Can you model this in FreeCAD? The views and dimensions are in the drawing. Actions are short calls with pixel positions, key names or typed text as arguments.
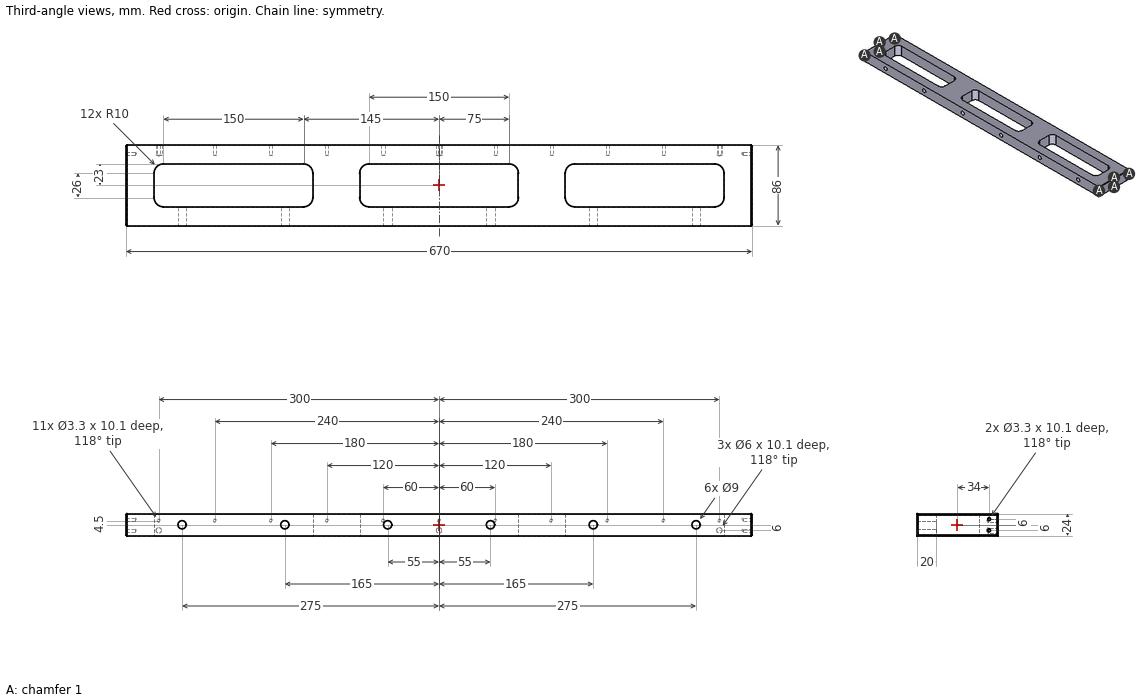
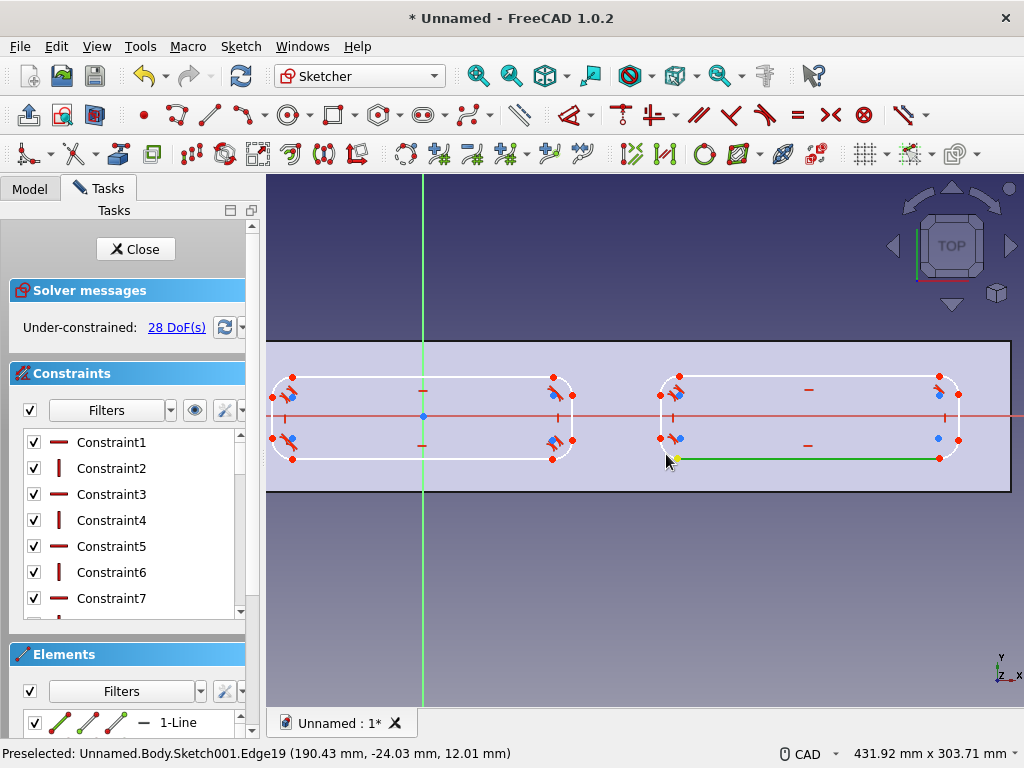
click(665, 452)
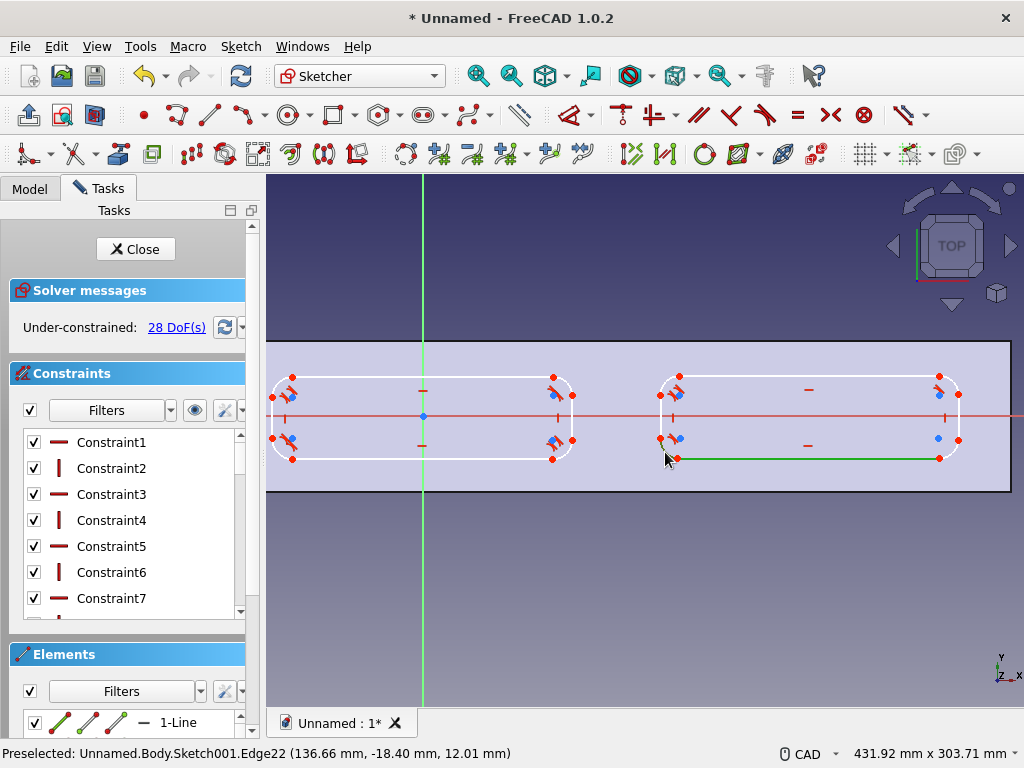
key(t)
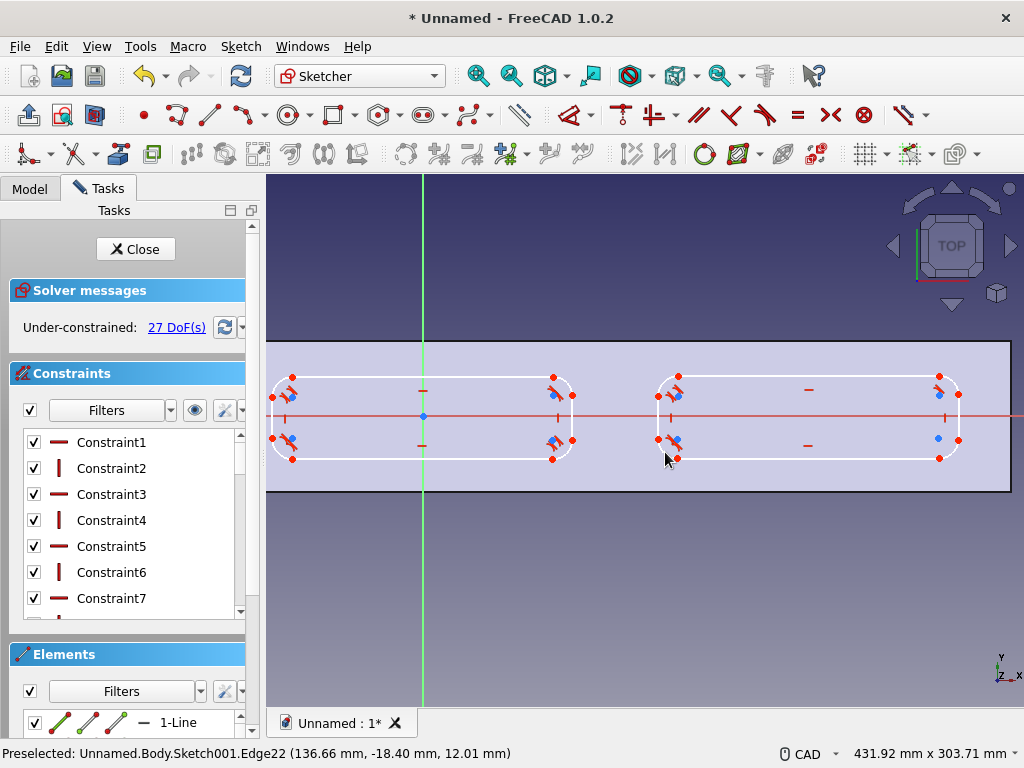
click(756, 459)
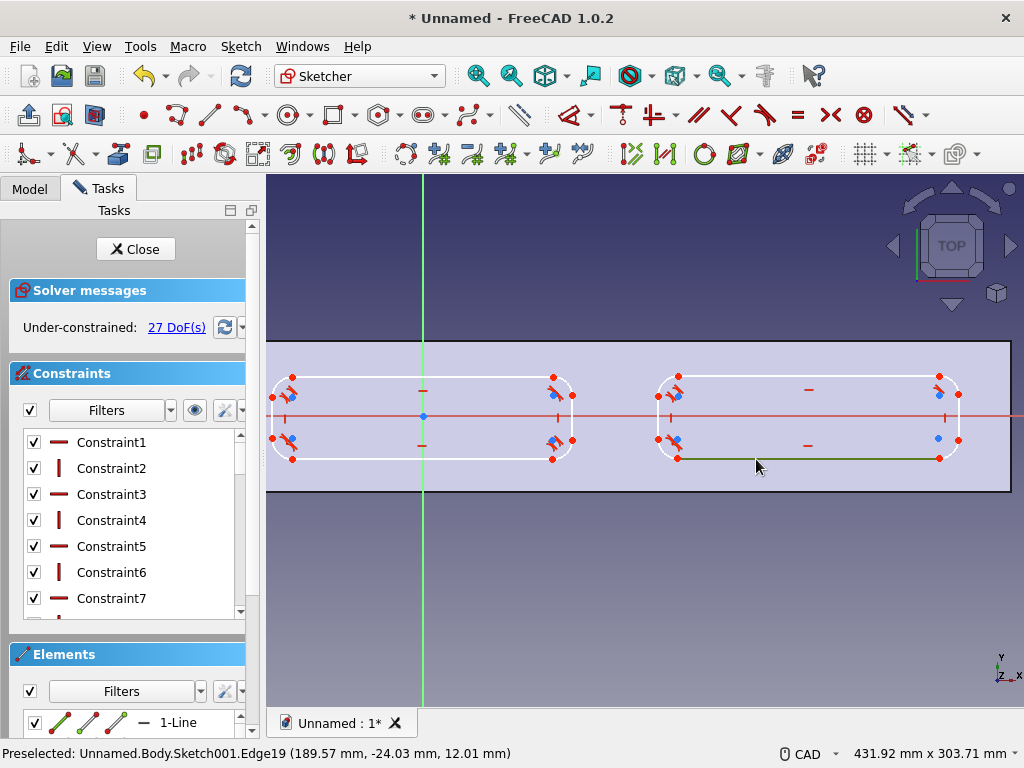
scroll(666, 454, down, 5)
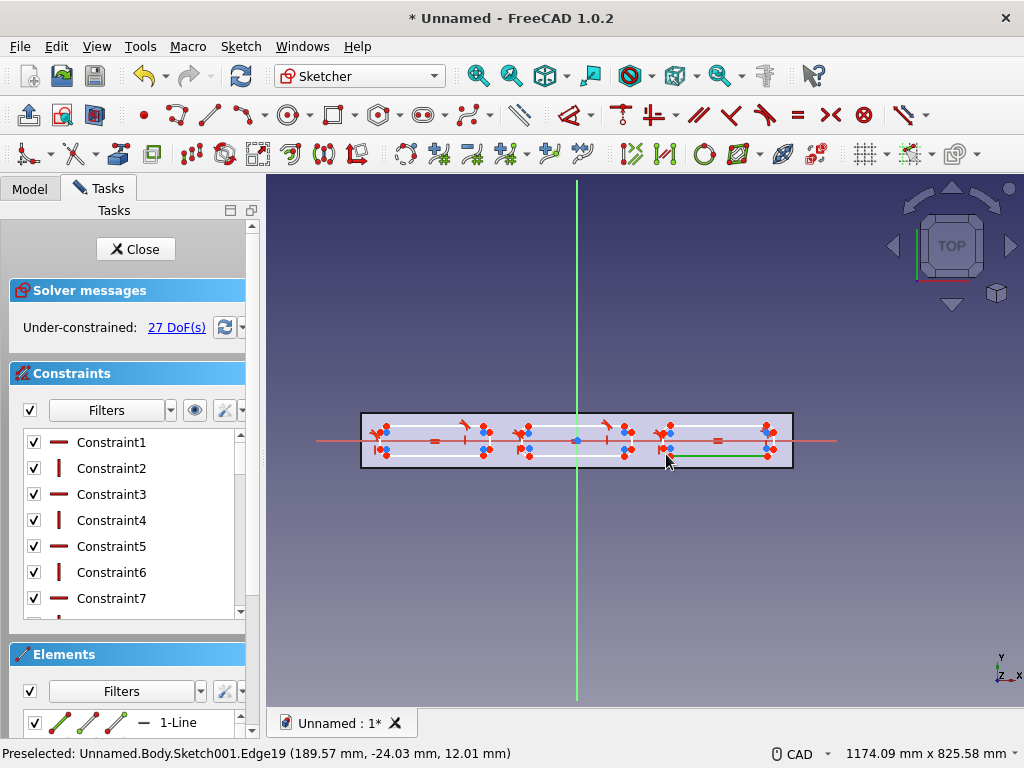
scroll(772, 454, up, 5)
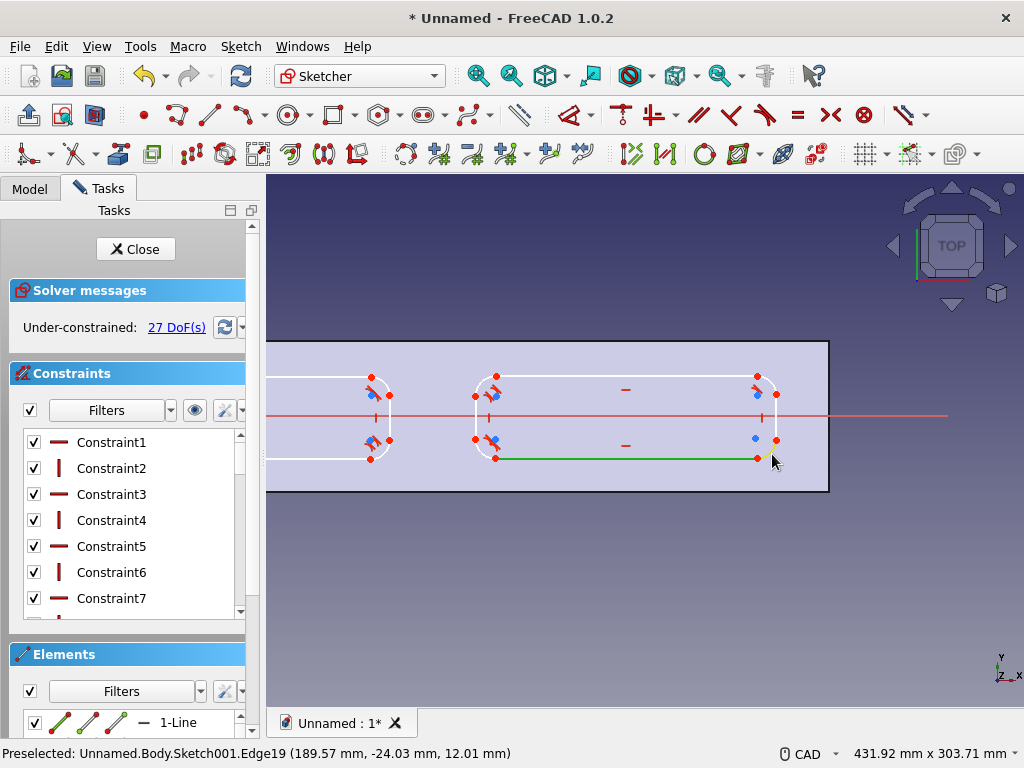
click(770, 453)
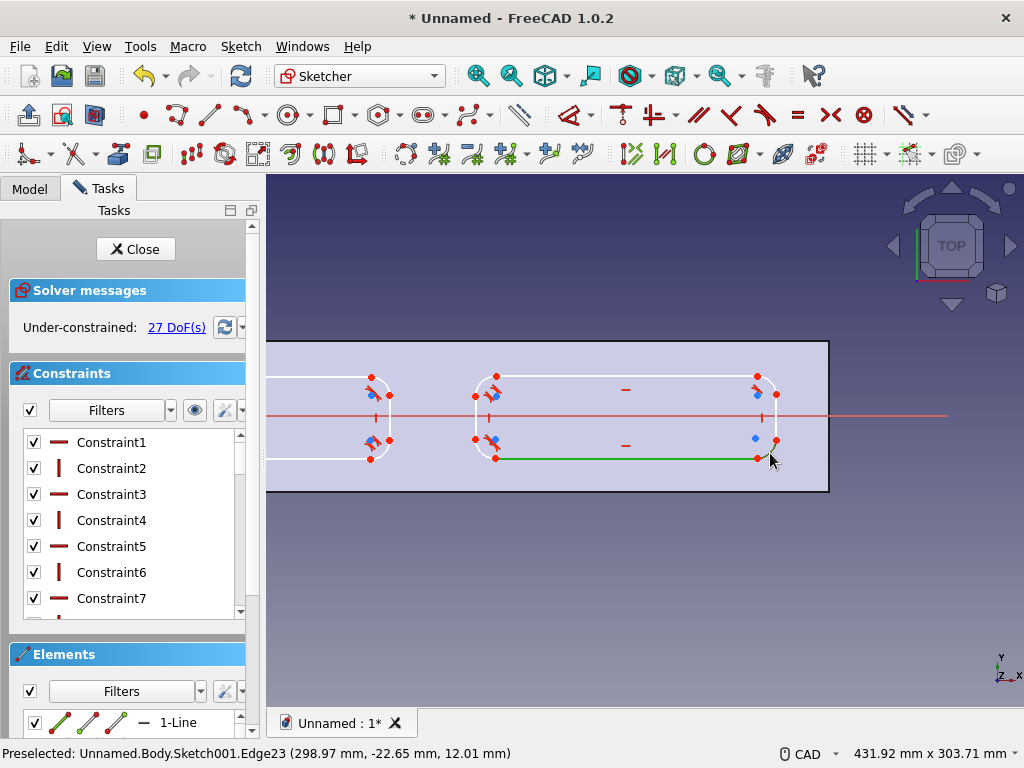
key(t)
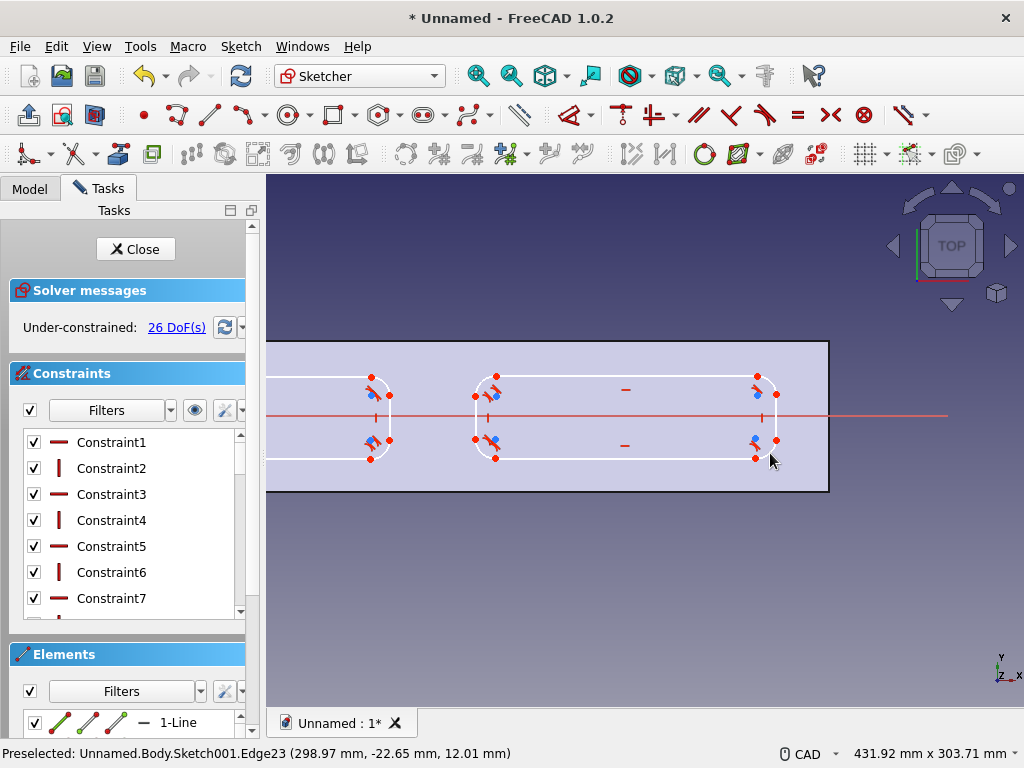
scroll(776, 427, up, 2)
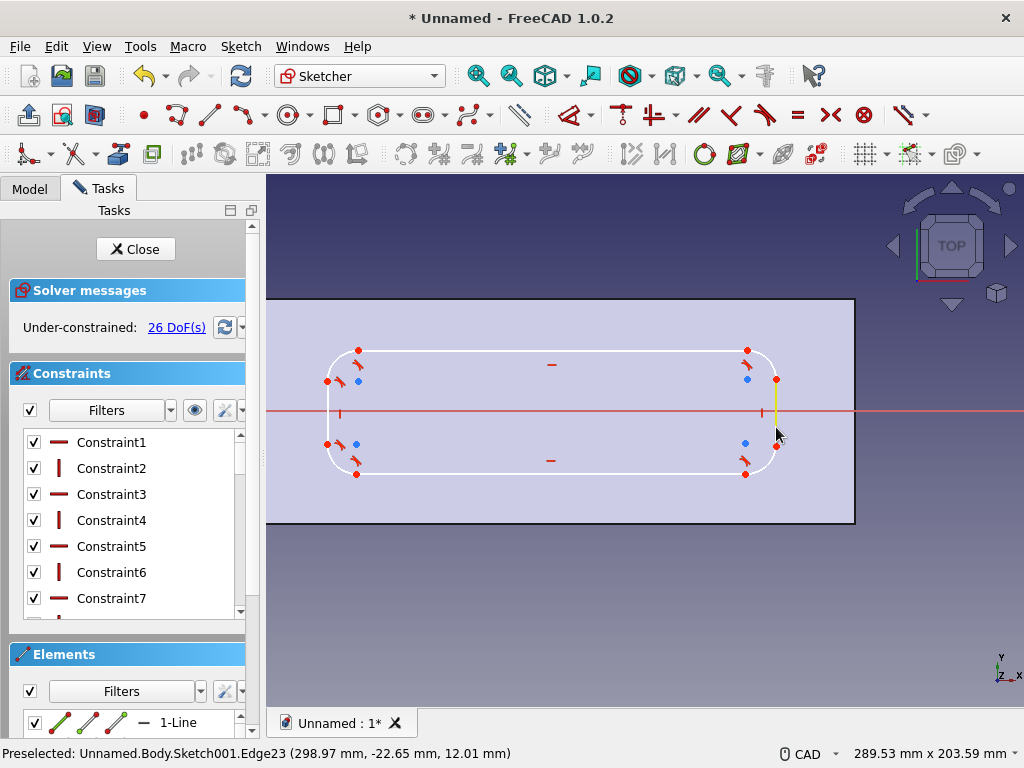
click(776, 426)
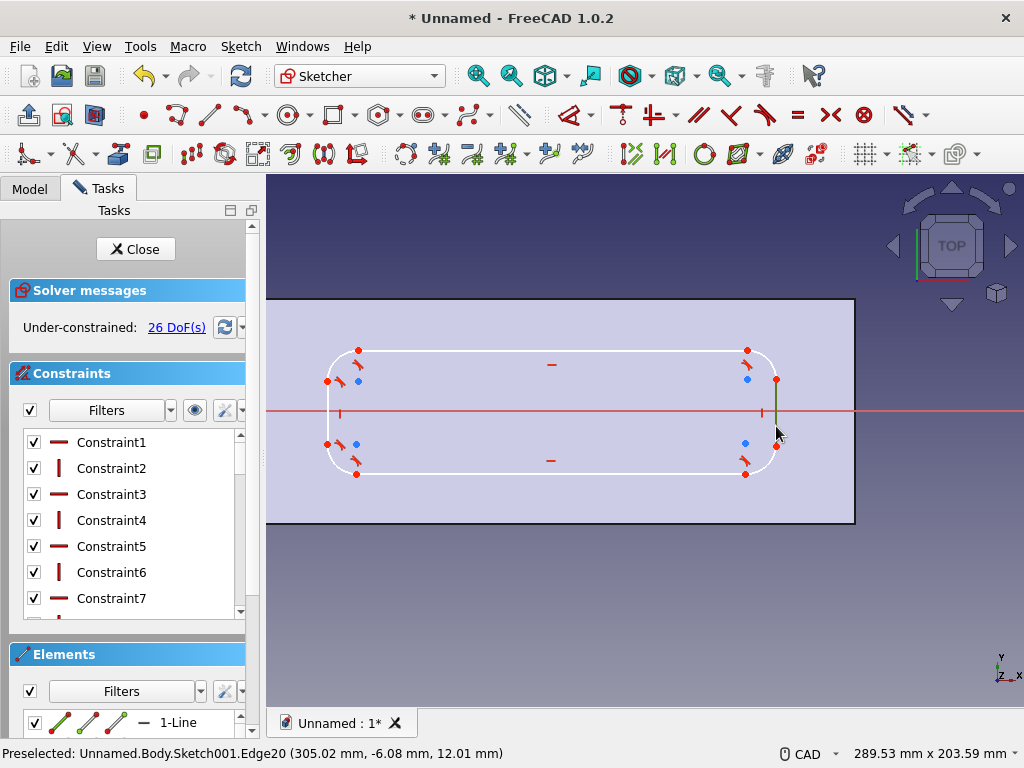
click(759, 471)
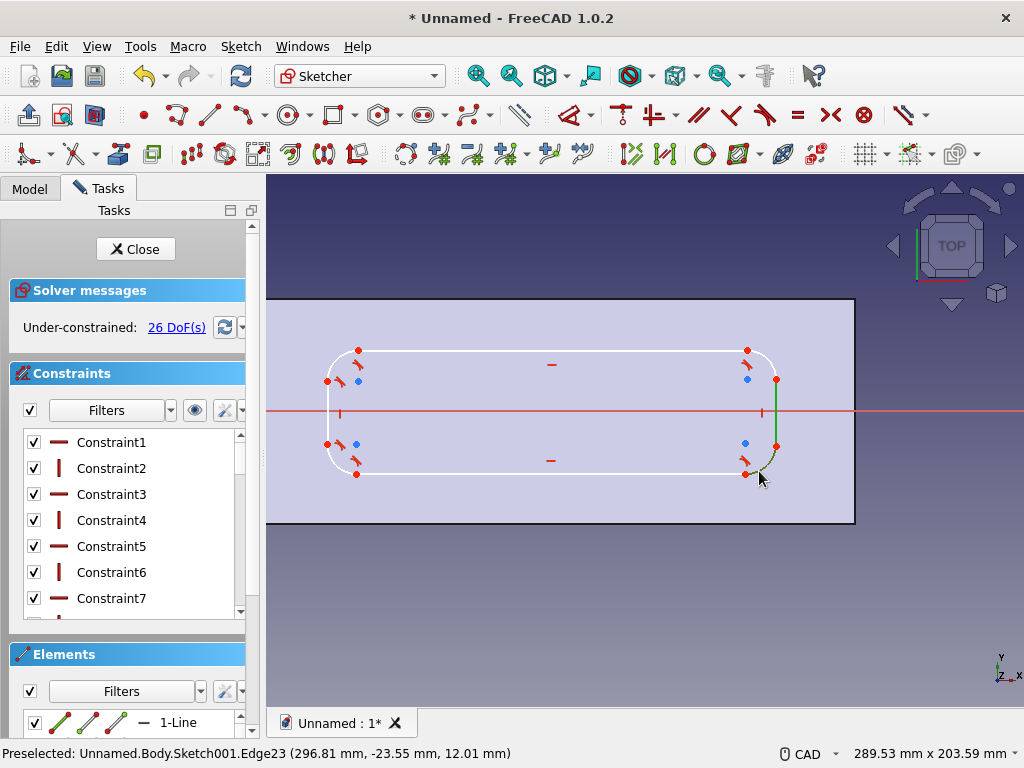
key(t)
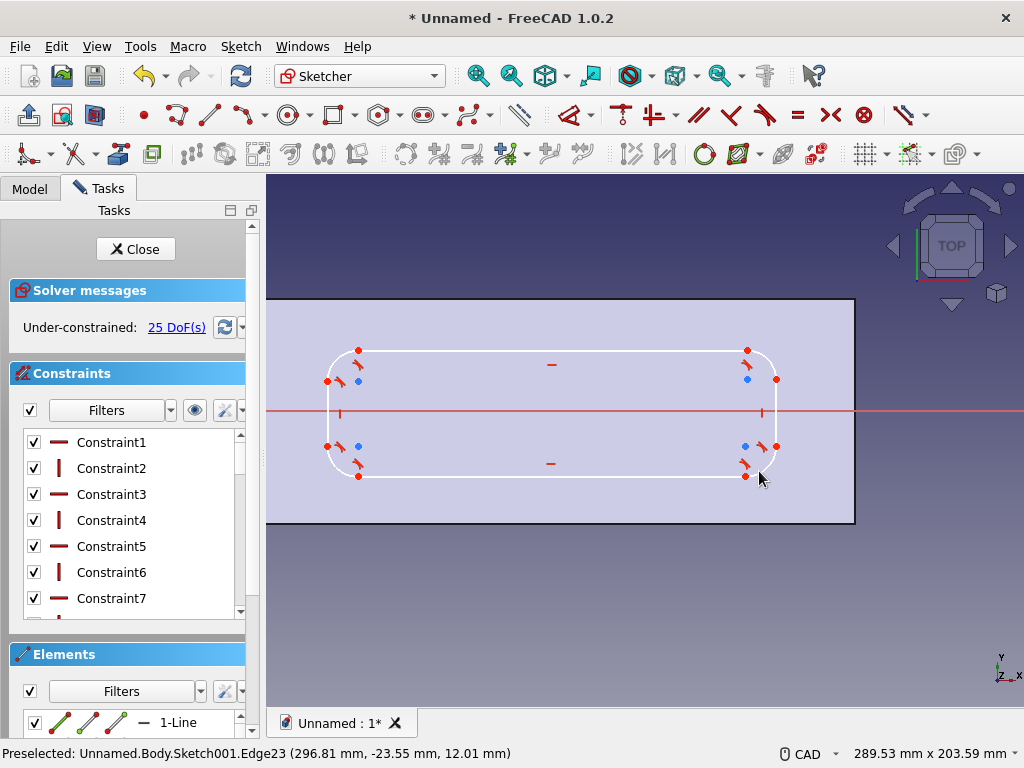
click(776, 426)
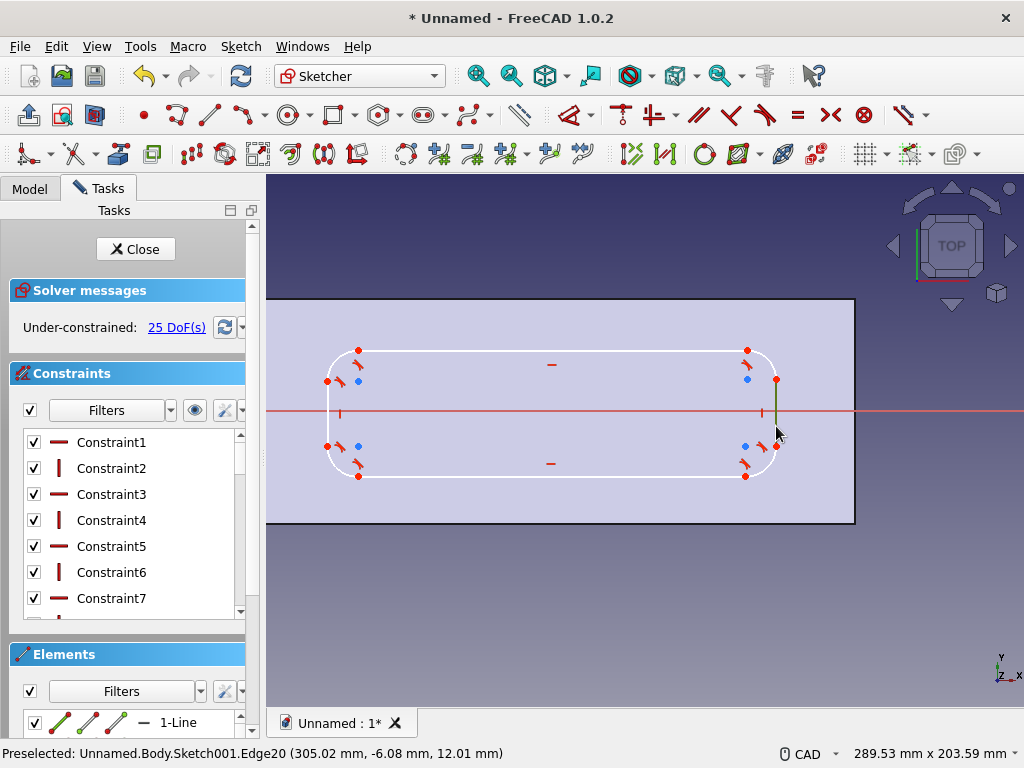
click(773, 366)